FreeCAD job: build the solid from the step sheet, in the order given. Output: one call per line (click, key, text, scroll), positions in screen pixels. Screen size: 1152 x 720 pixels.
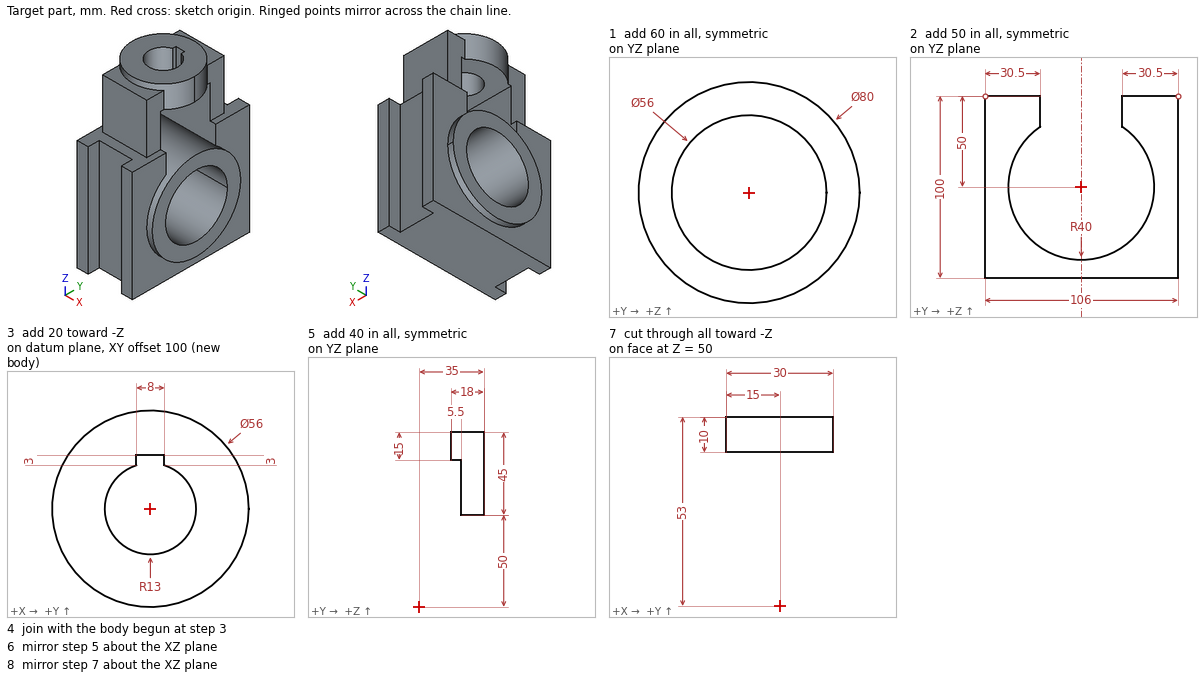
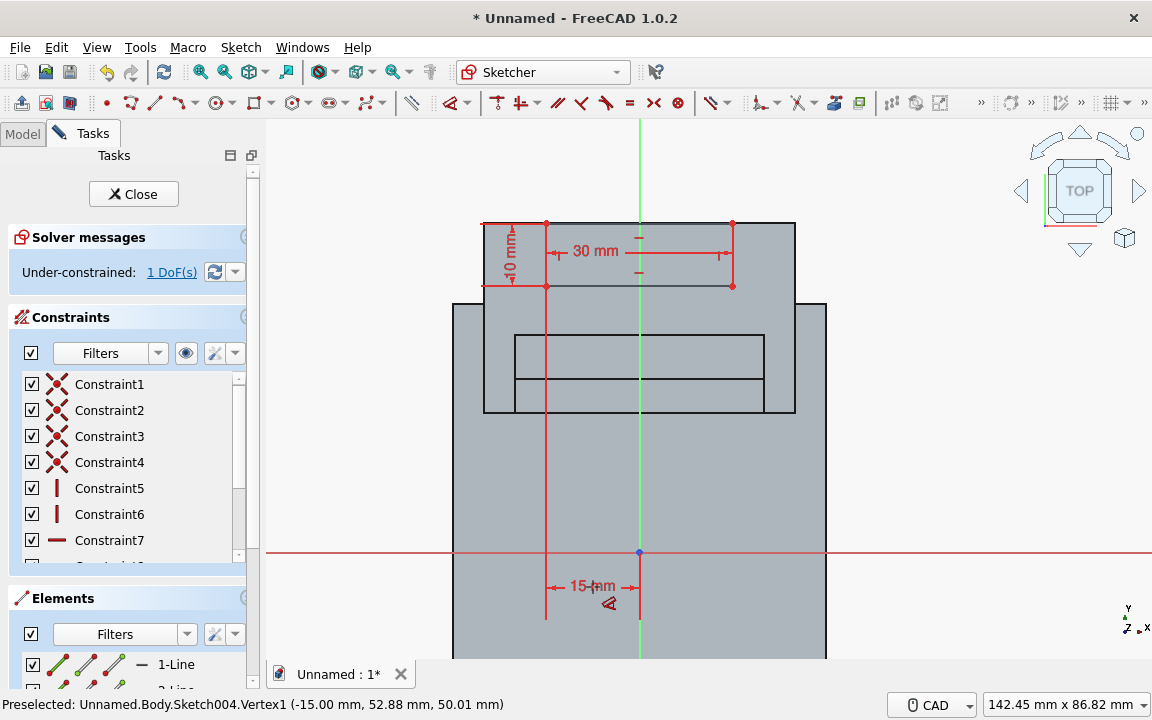
click(546, 224)
click(512, 388)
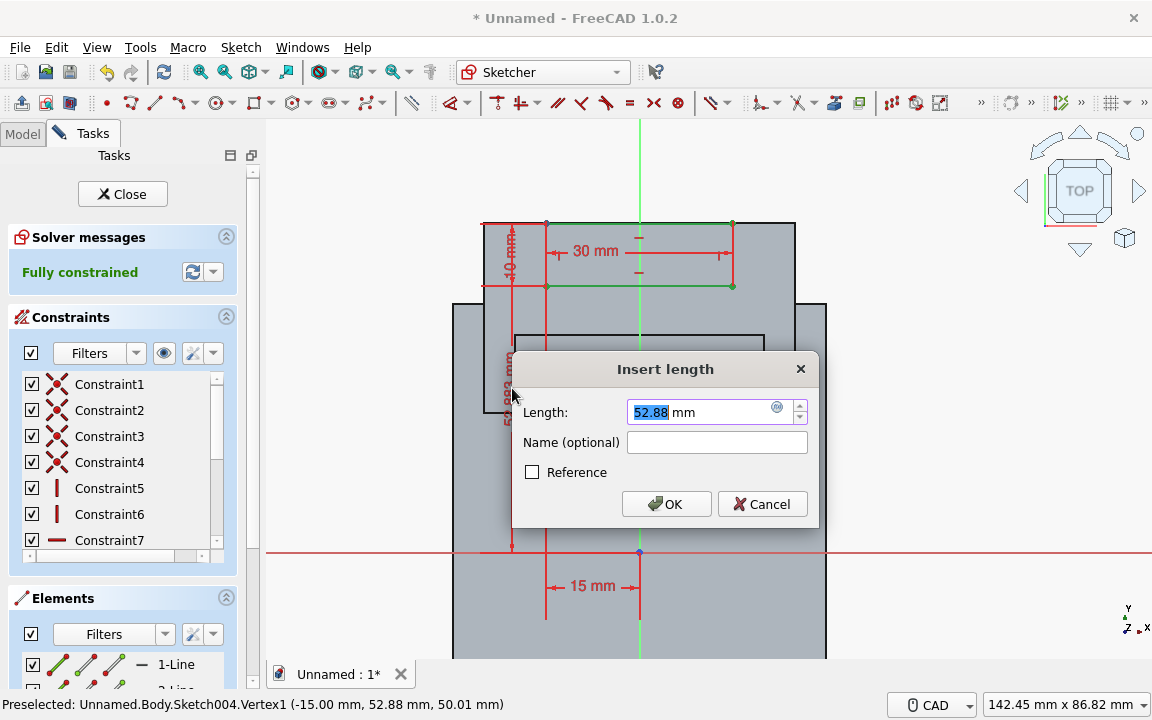
text(53)
key(Return)
key(Escape)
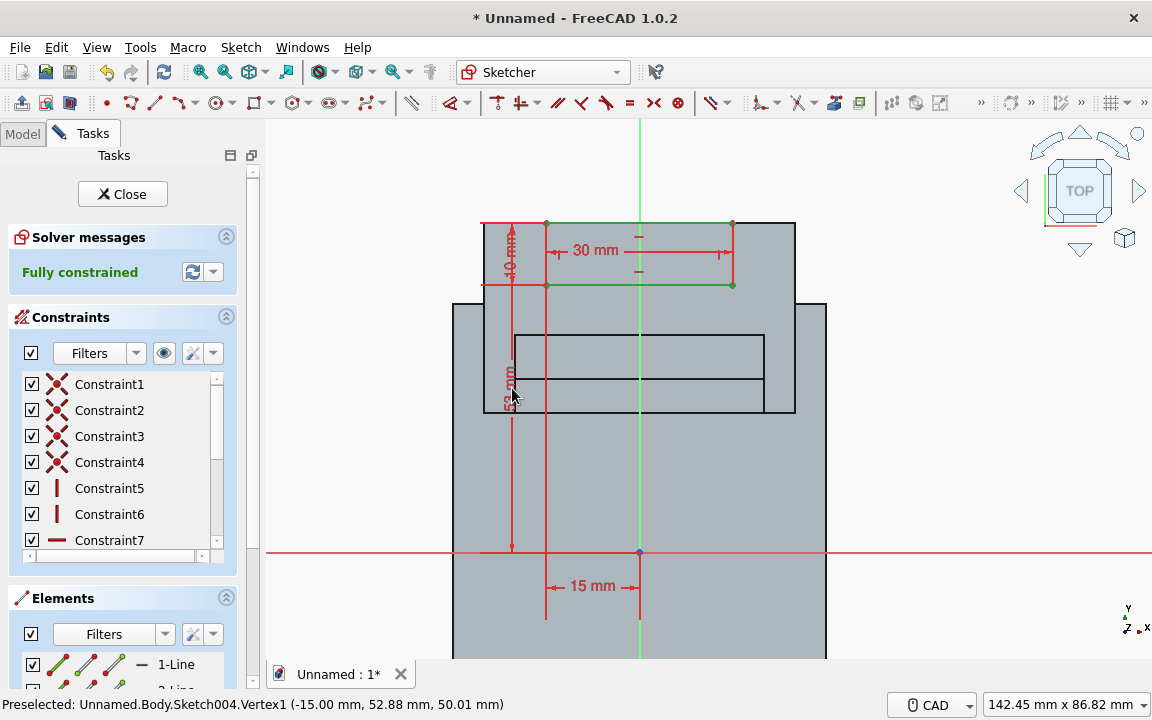
click(123, 194)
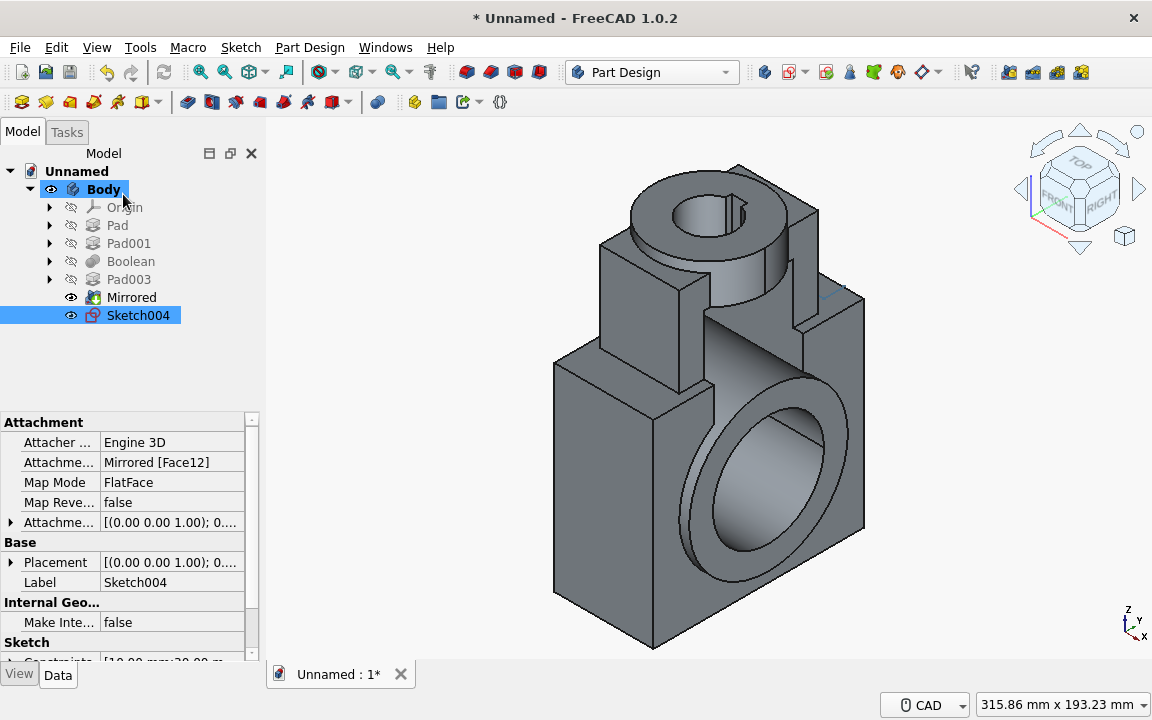
click(188, 102)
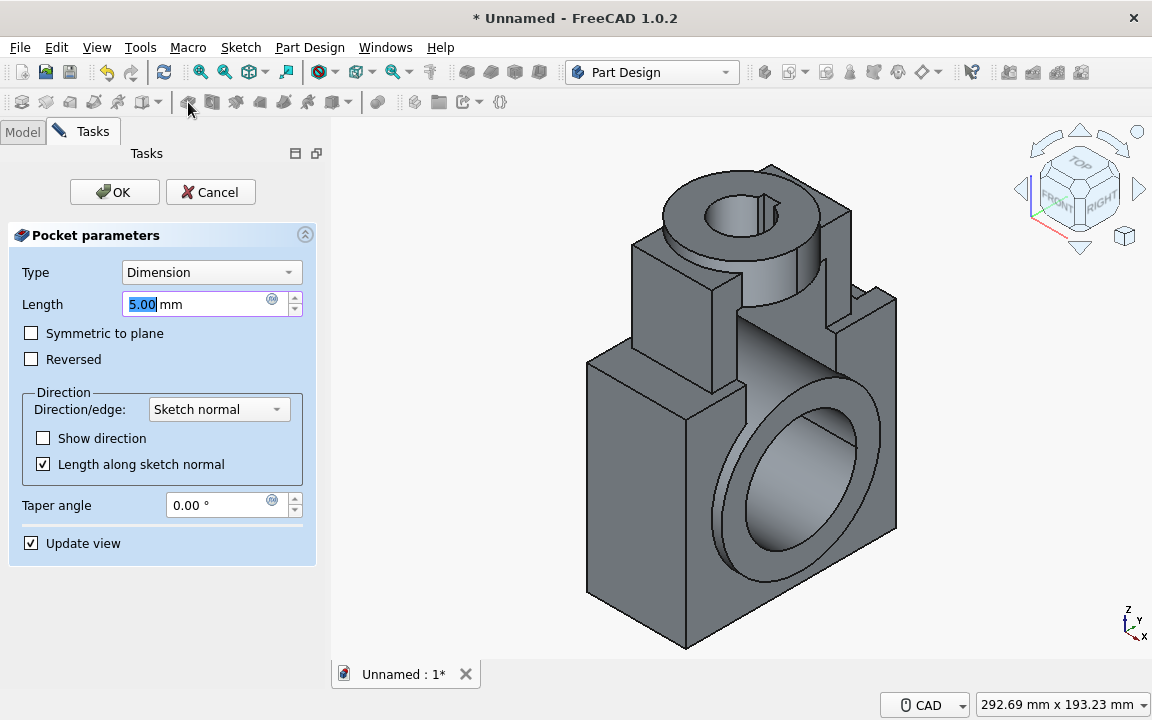
click(212, 272)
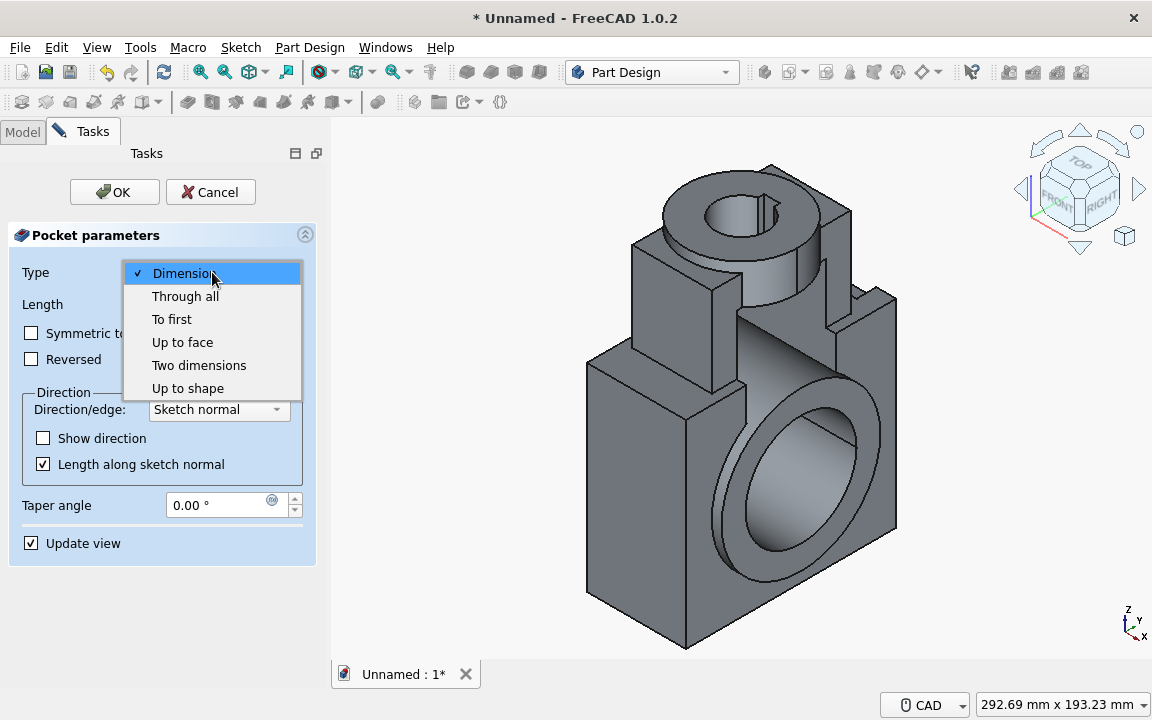
click(212, 296)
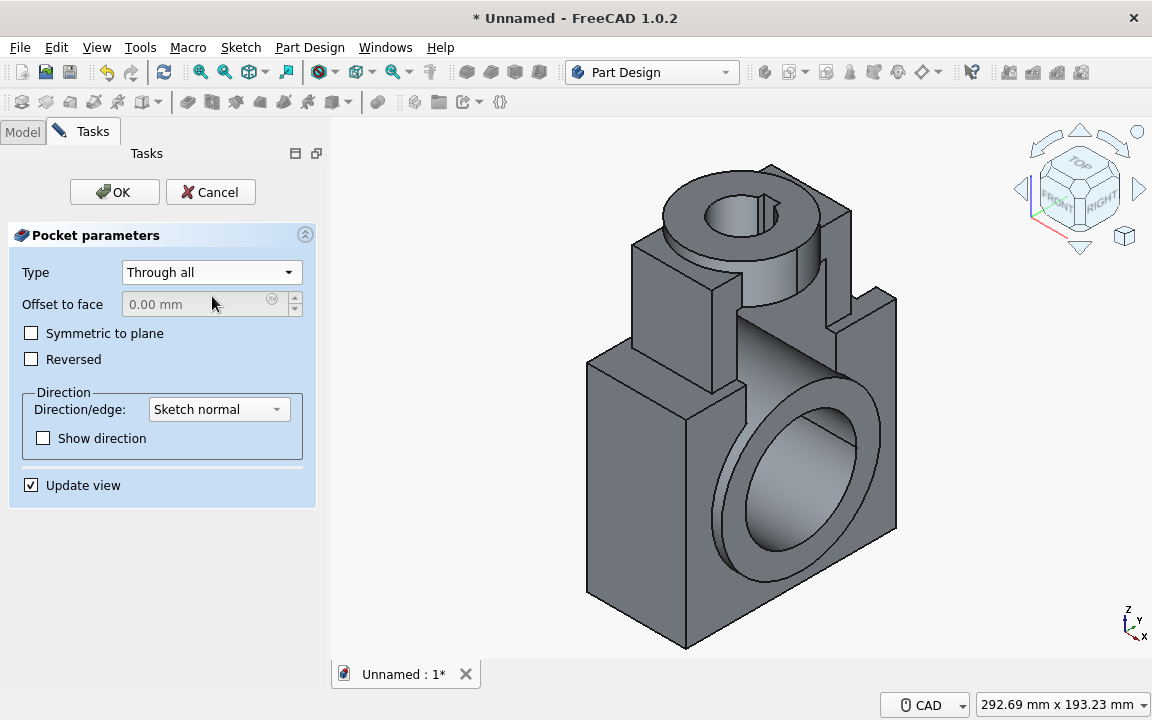
click(115, 192)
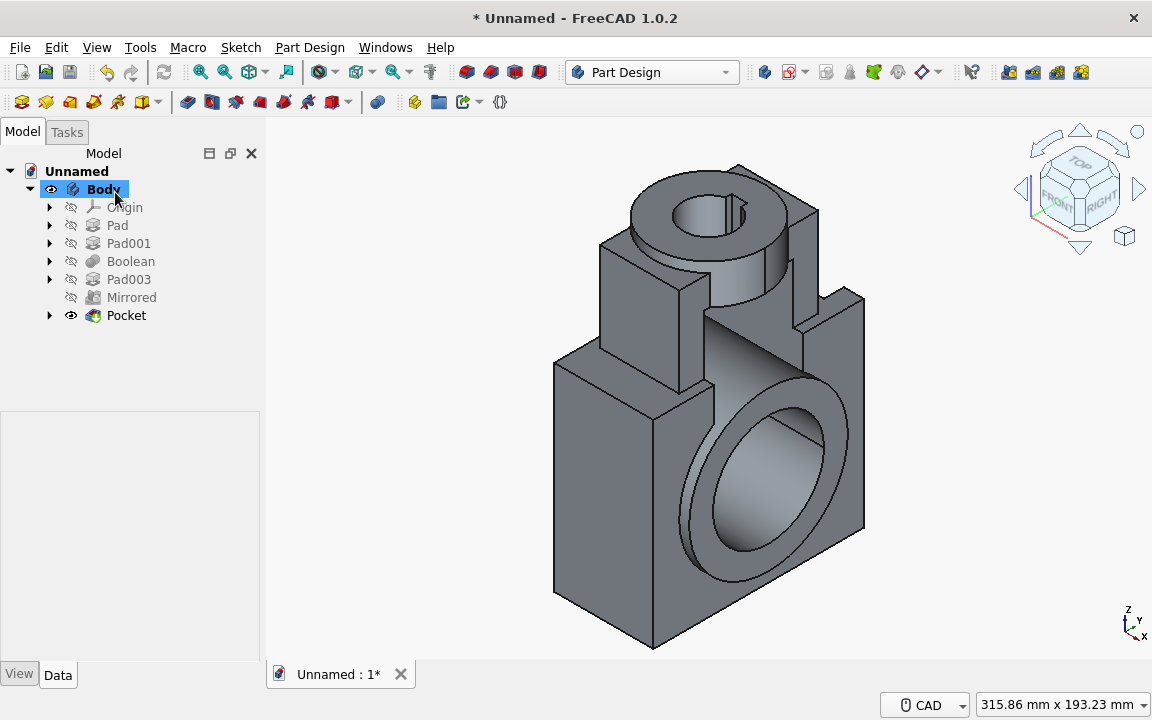
click(116, 315)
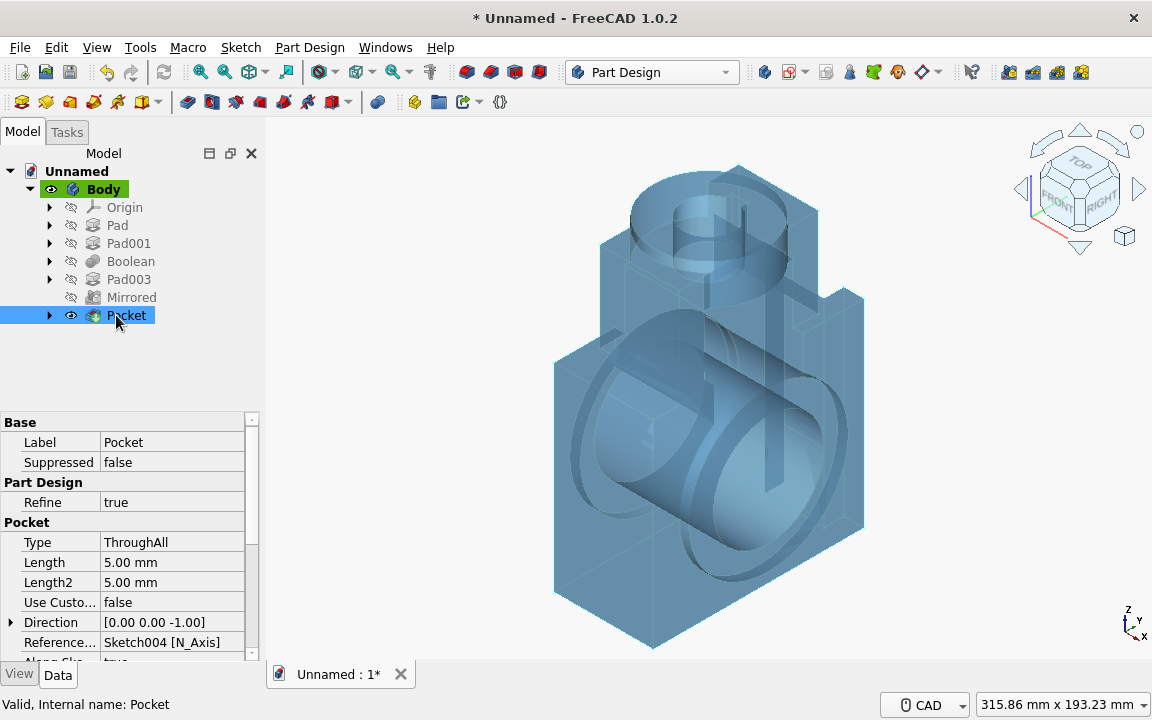
click(1010, 72)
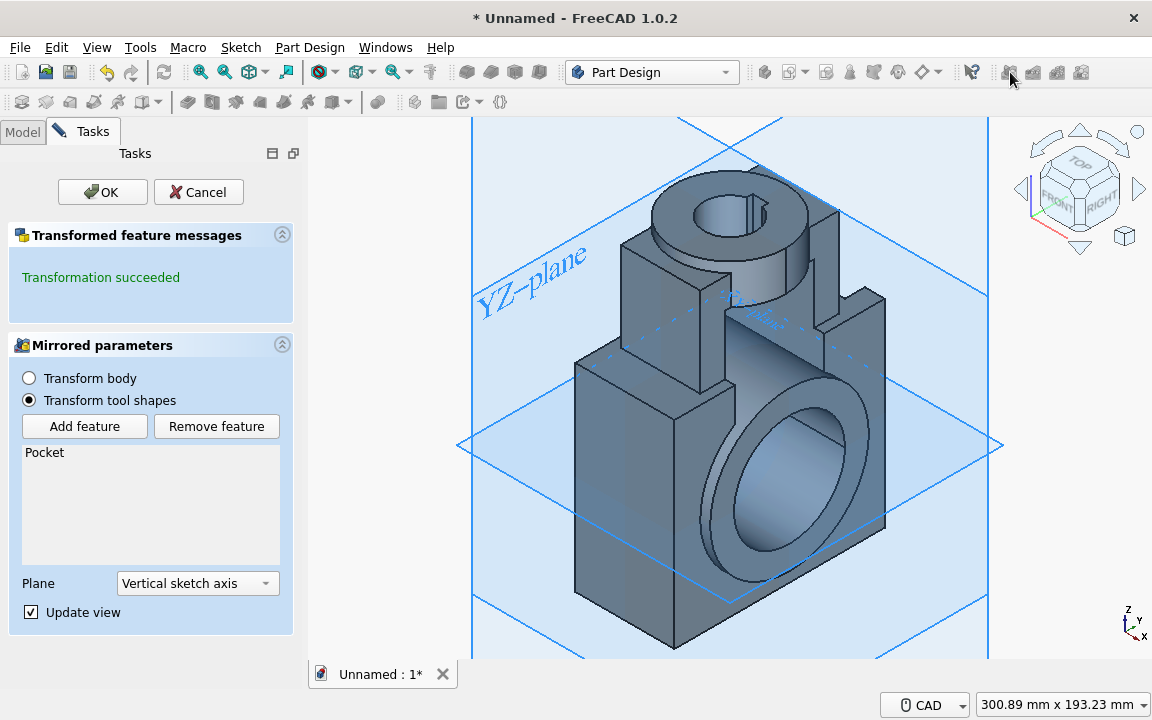
click(198, 584)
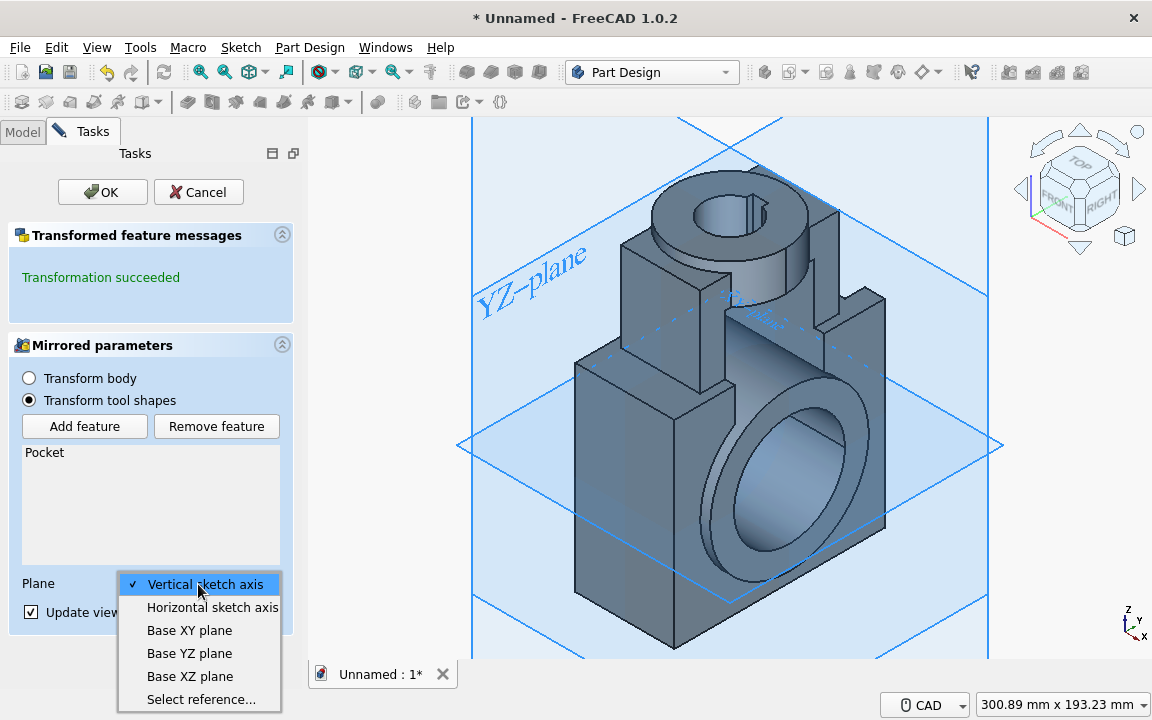
click(198, 676)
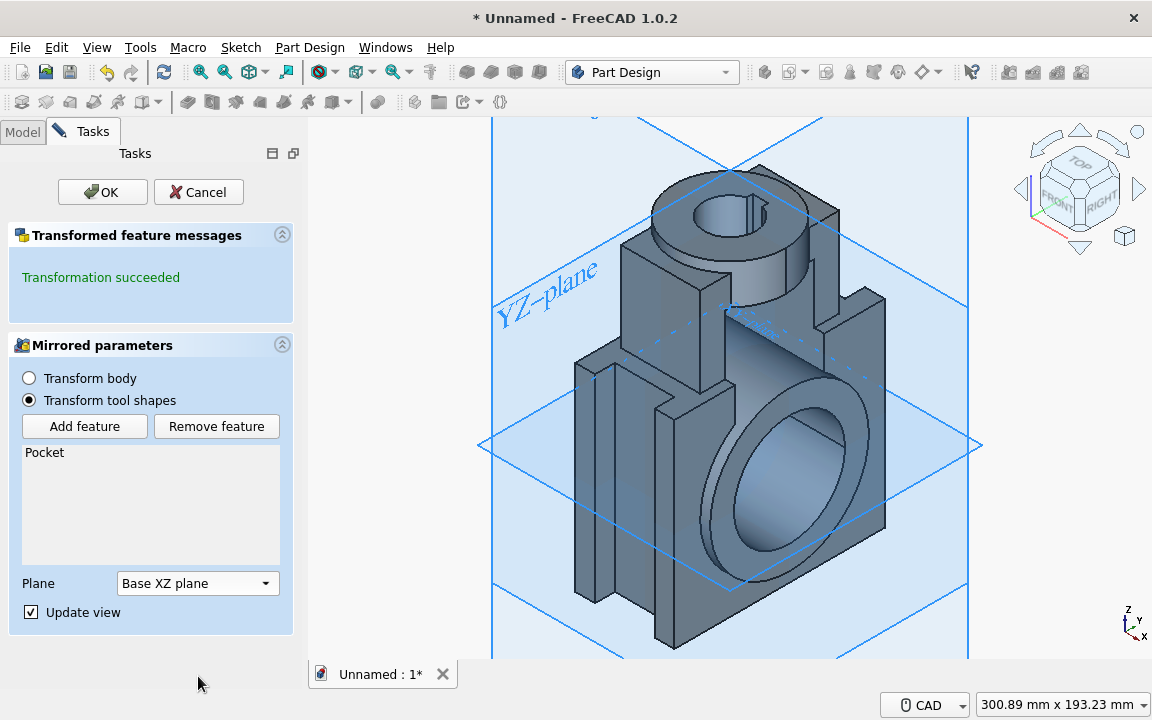
click(103, 192)